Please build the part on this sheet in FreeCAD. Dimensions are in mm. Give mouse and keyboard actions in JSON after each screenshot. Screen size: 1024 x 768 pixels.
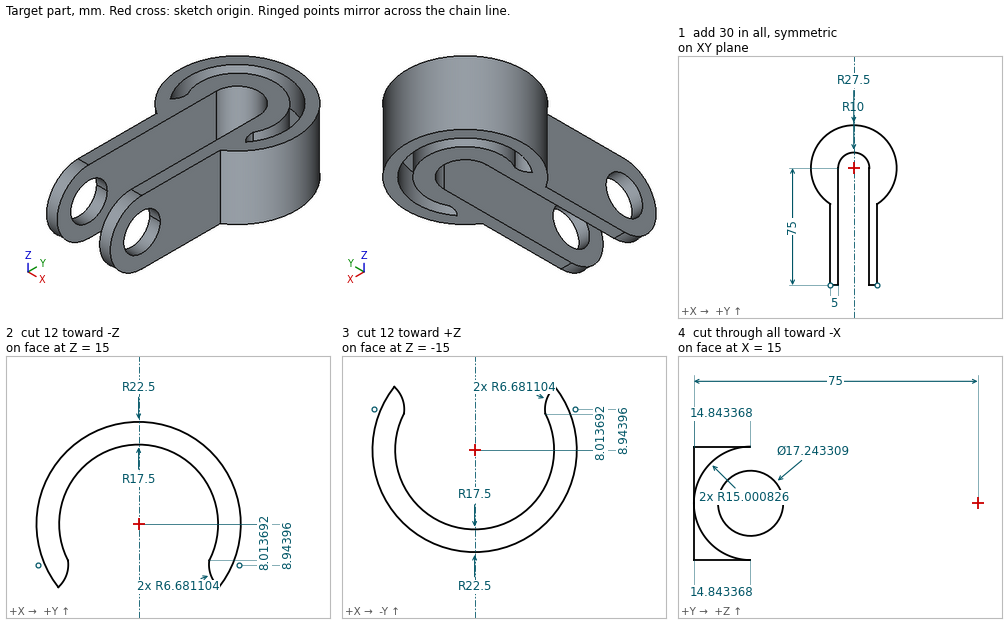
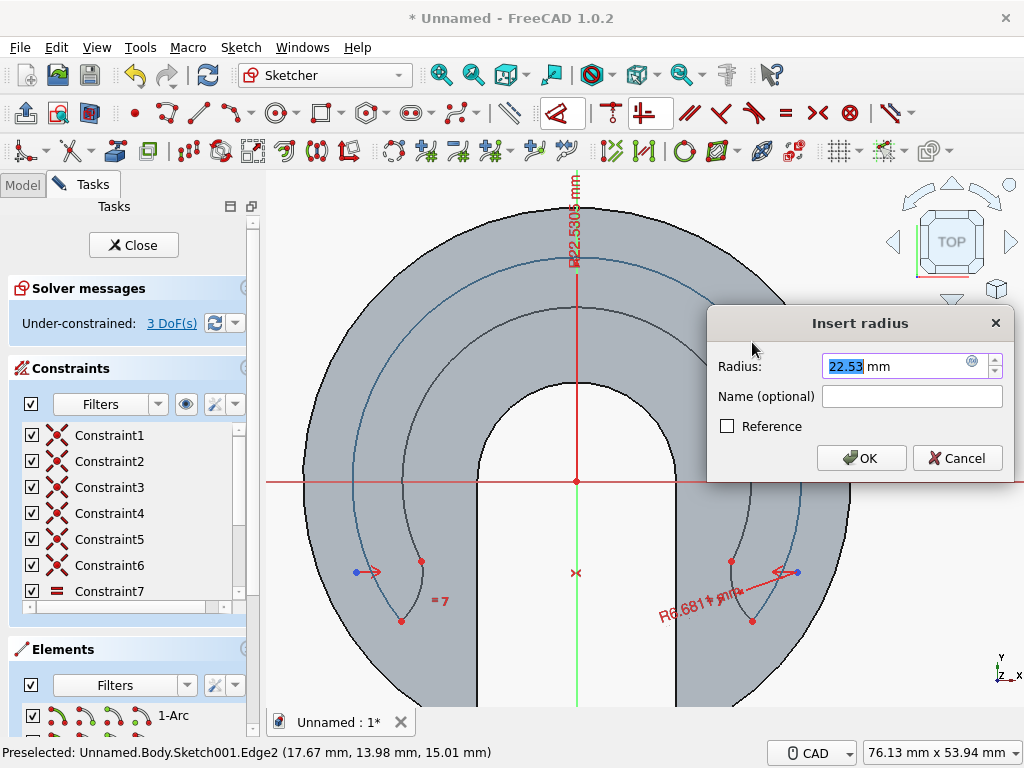
{"action": "type", "text": "22.5"}
{"action": "key", "text": "Return"}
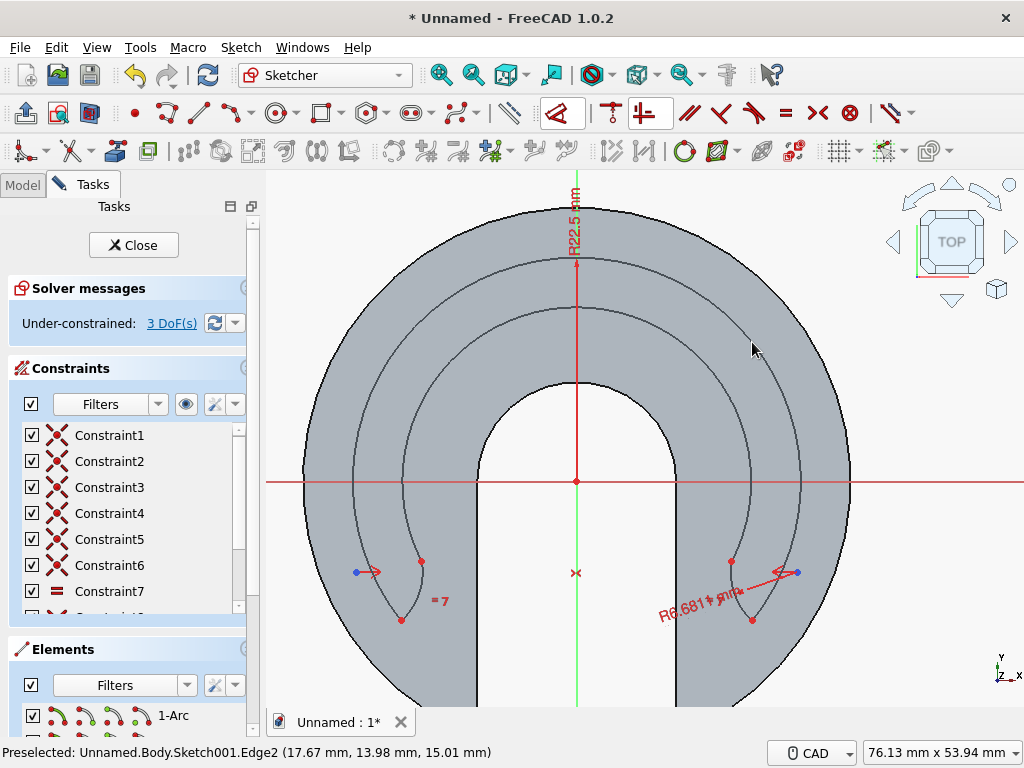
{"action": "left_click", "coordinate": [704, 363]}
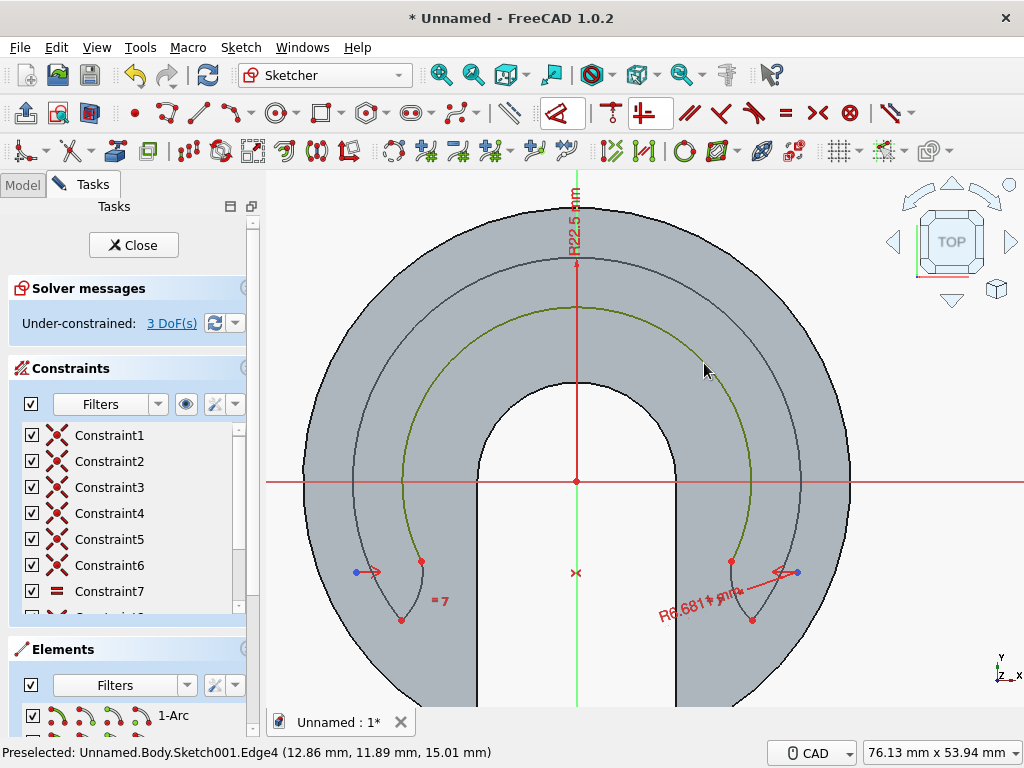
{"action": "key", "text": "k r"}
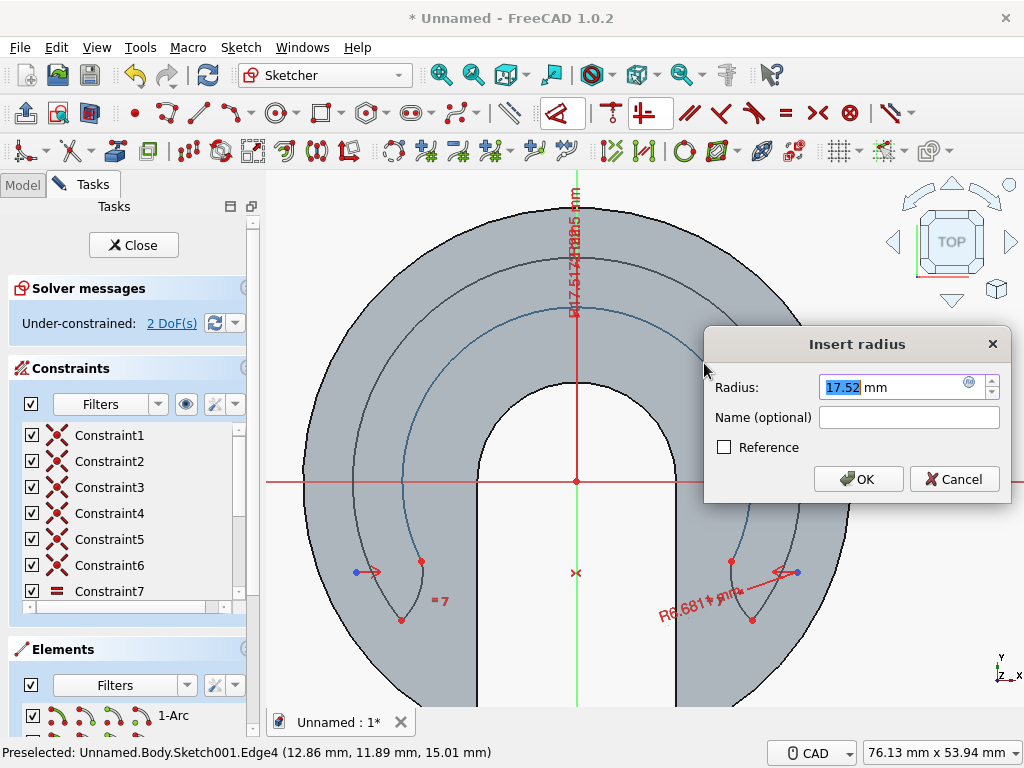
{"action": "type", "text": "17.5"}
{"action": "key", "text": "Return"}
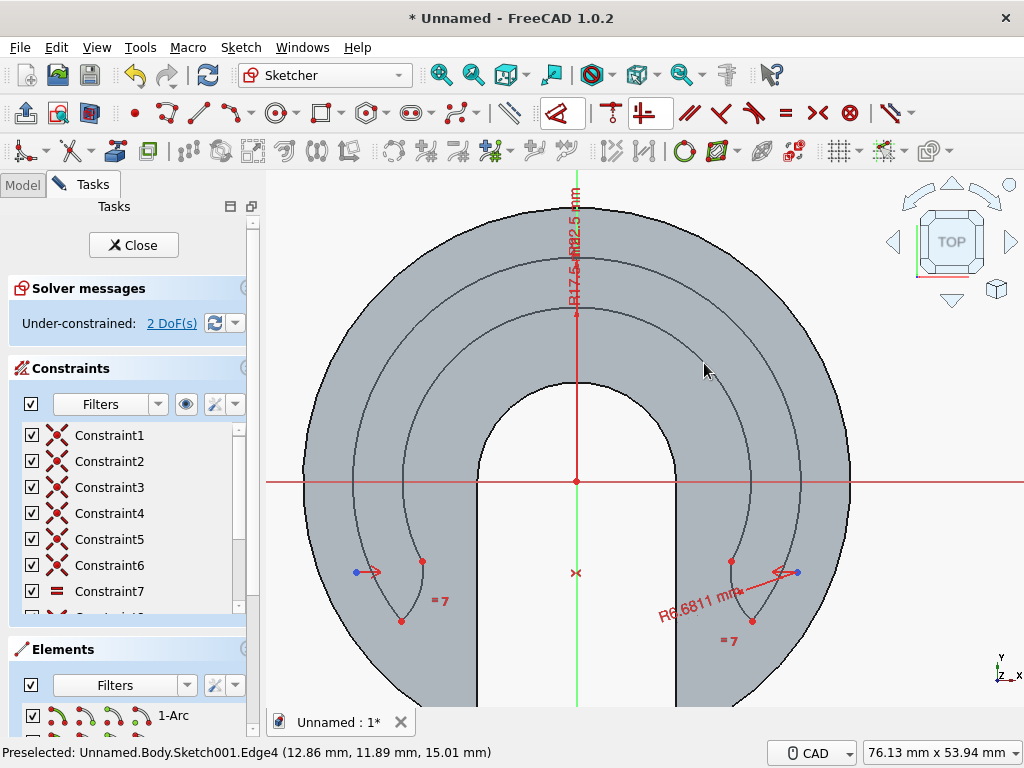
{"action": "left_click", "coordinate": [797, 572]}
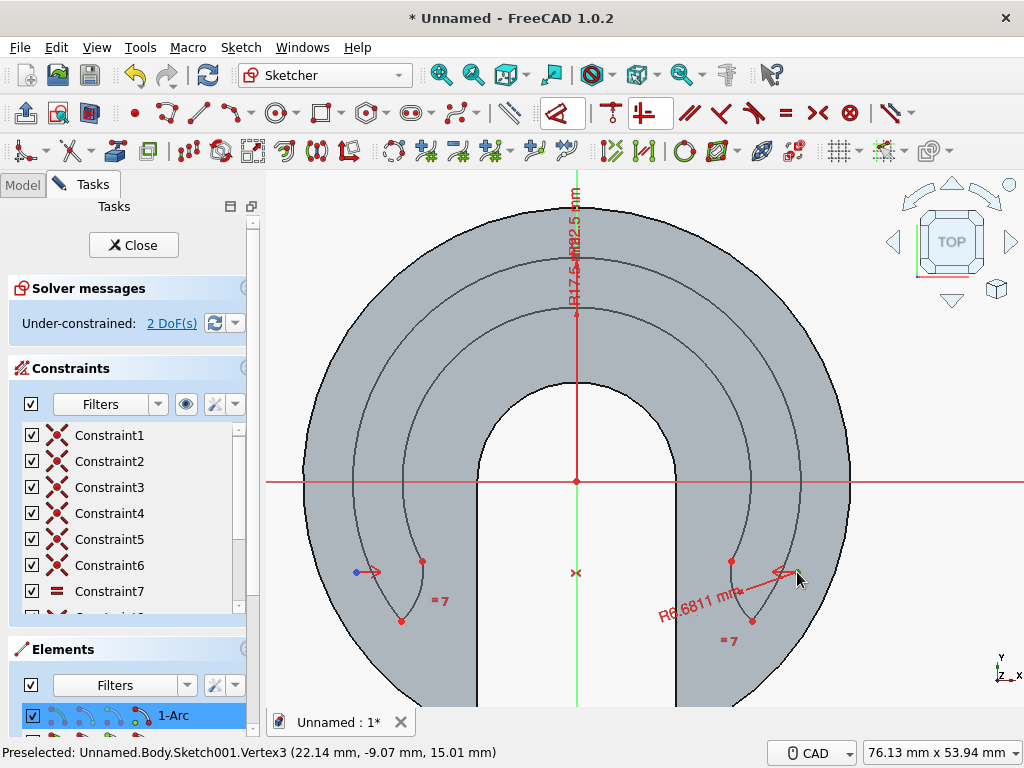
{"action": "key", "text": "i"}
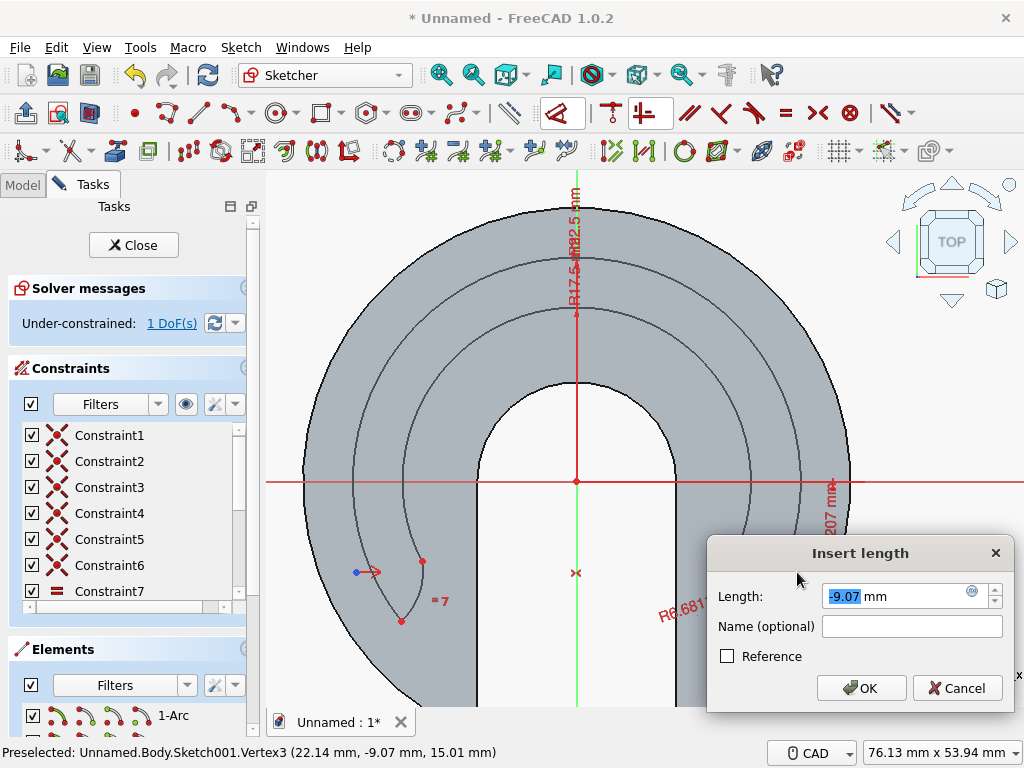
{"action": "type", "text": "-8.94396"}
{"action": "key", "text": "Return"}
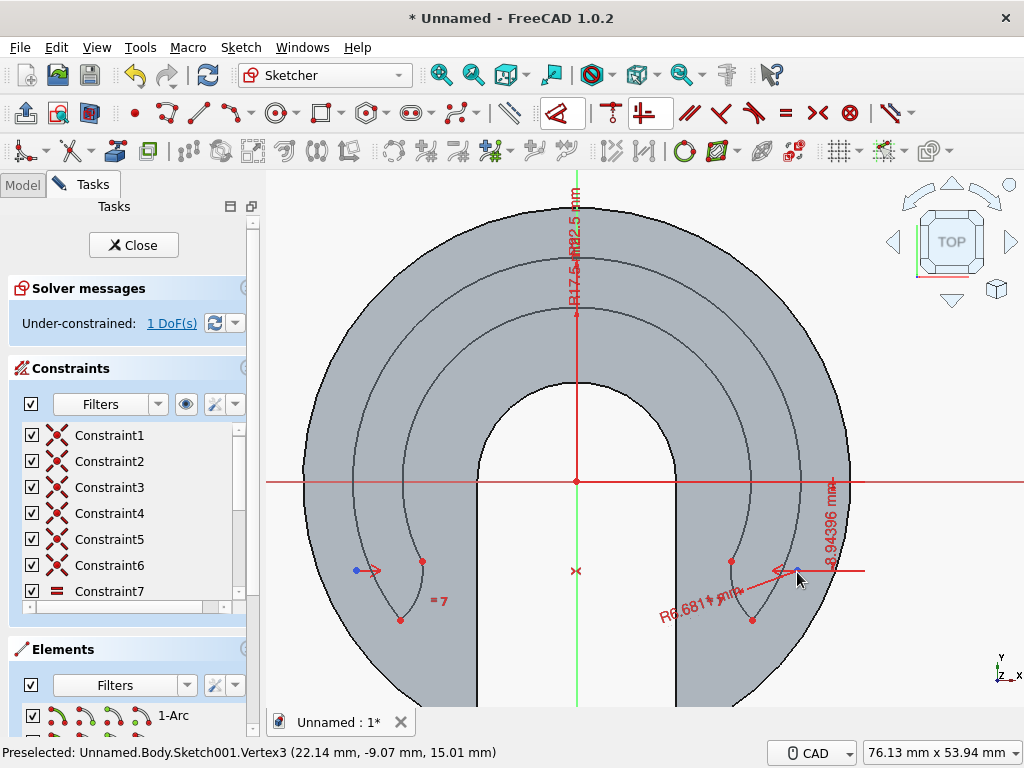
{"action": "left_click", "coordinate": [731, 562]}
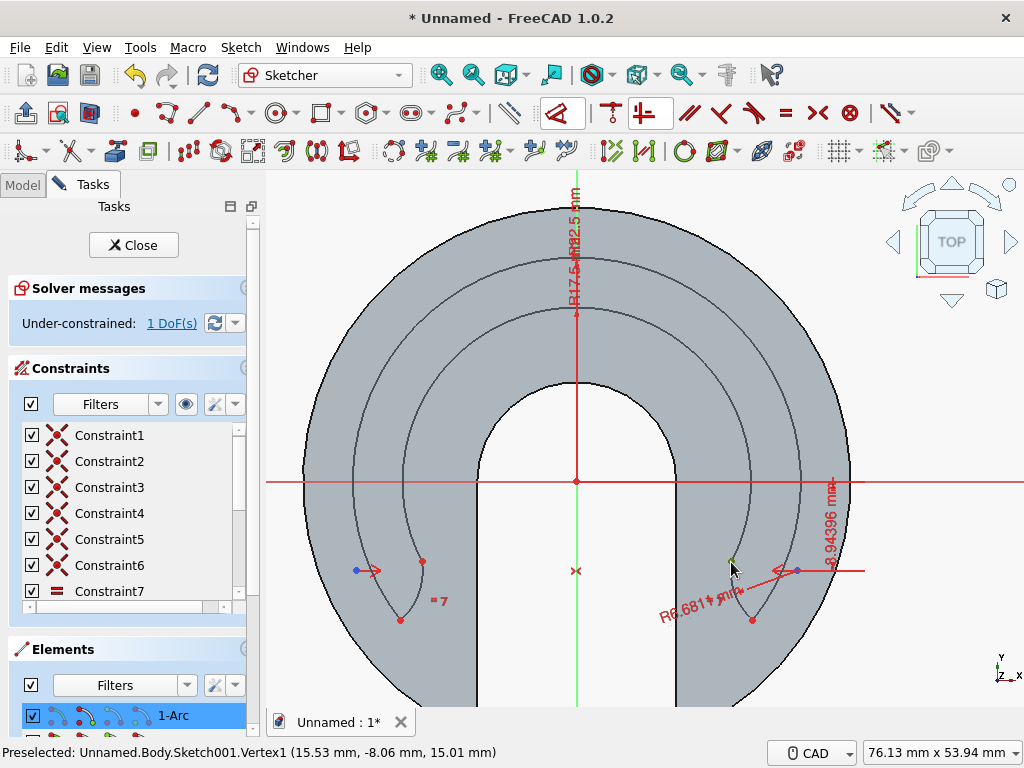
{"action": "key", "text": "i"}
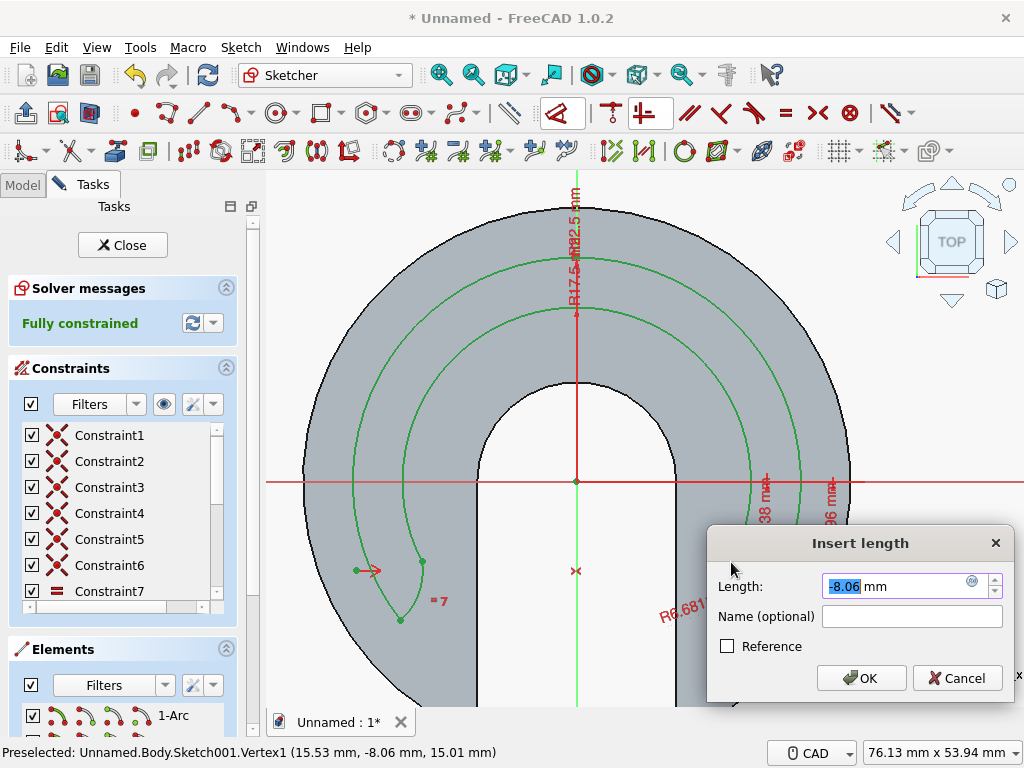
{"action": "type", "text": "-8.013692"}
{"action": "key", "text": "Return"}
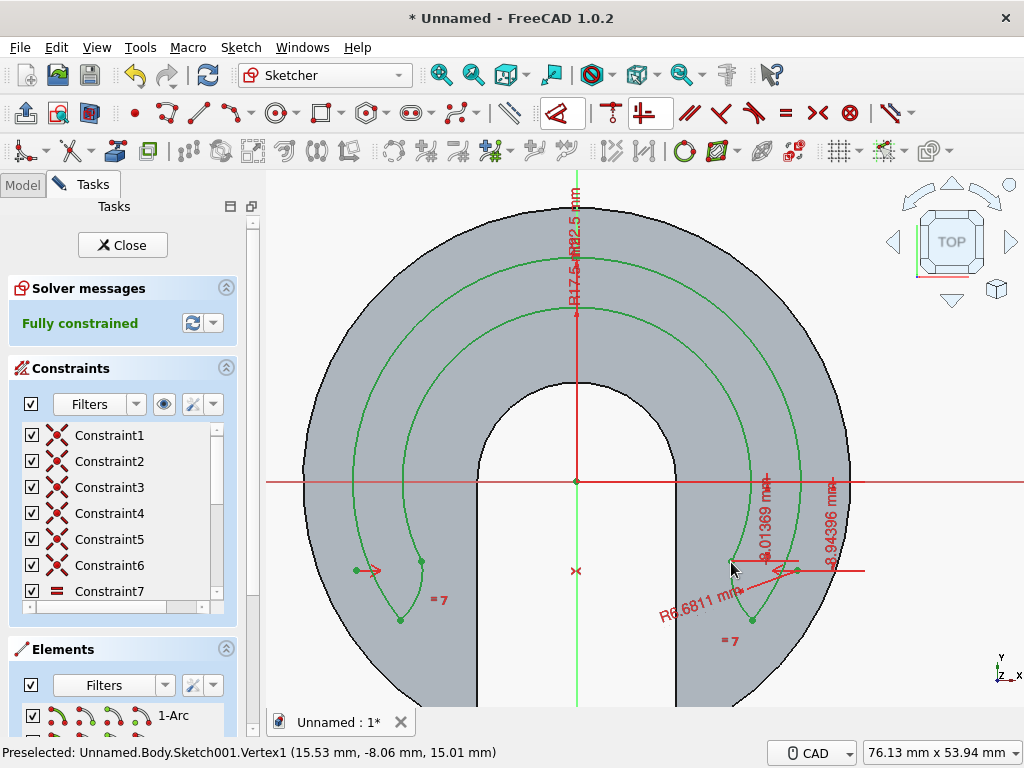
{"action": "left_click", "coordinate": [123, 245]}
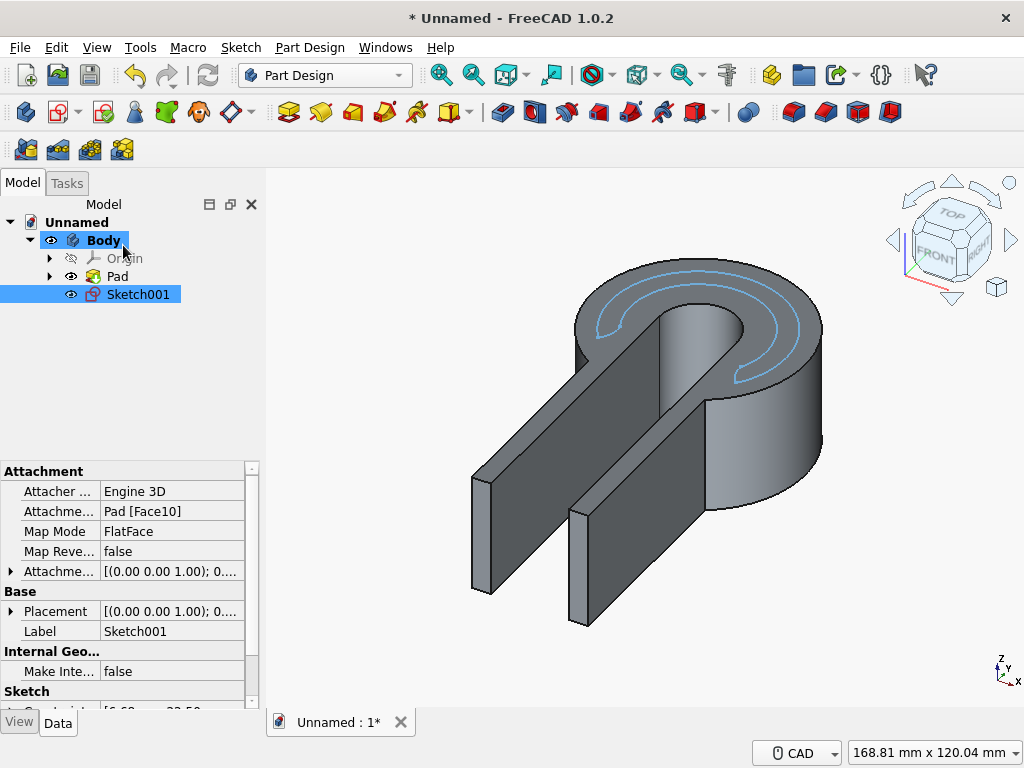
{"action": "left_click", "coordinate": [504, 112]}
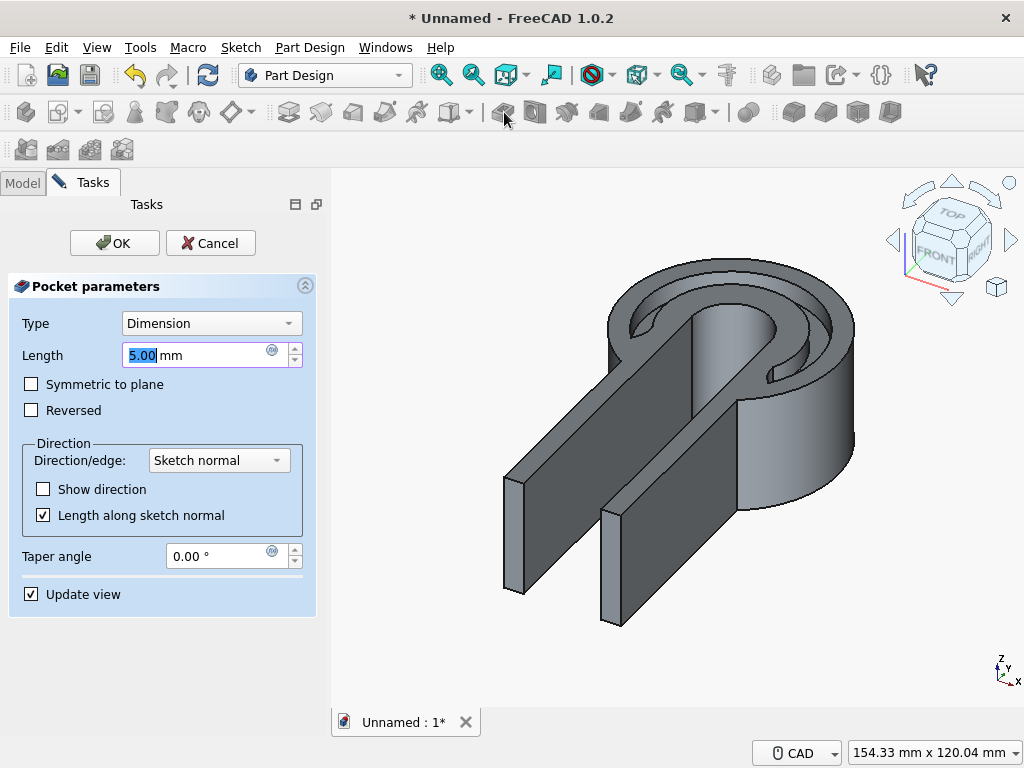
{"action": "type", "text": "12"}
{"action": "key", "text": "Tab"}